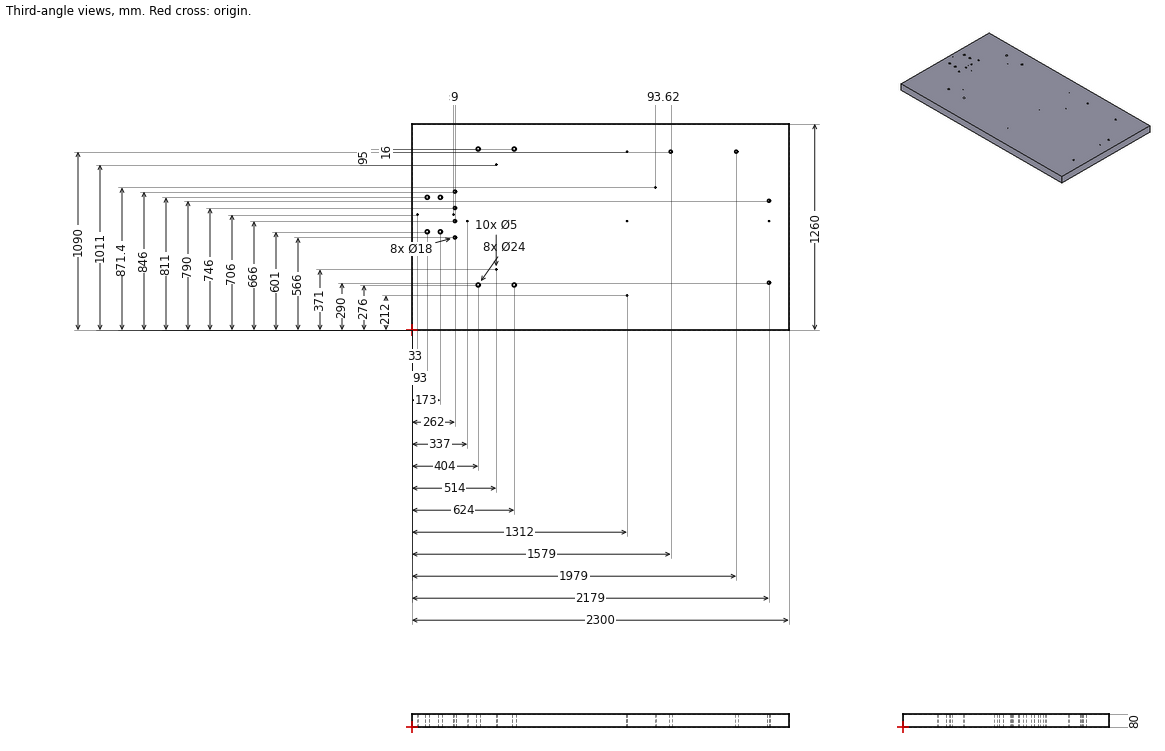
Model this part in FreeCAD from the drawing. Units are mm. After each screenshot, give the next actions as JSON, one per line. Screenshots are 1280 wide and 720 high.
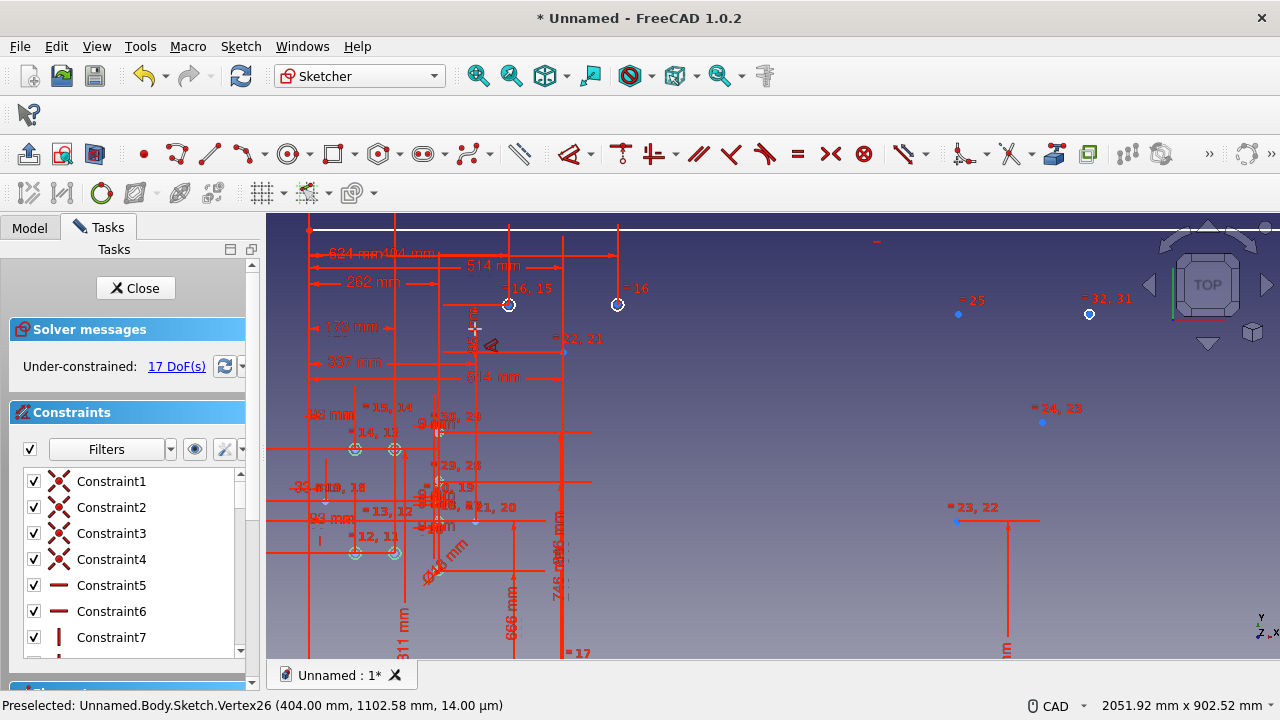
{"action": "left_click", "coordinate": [563, 352]}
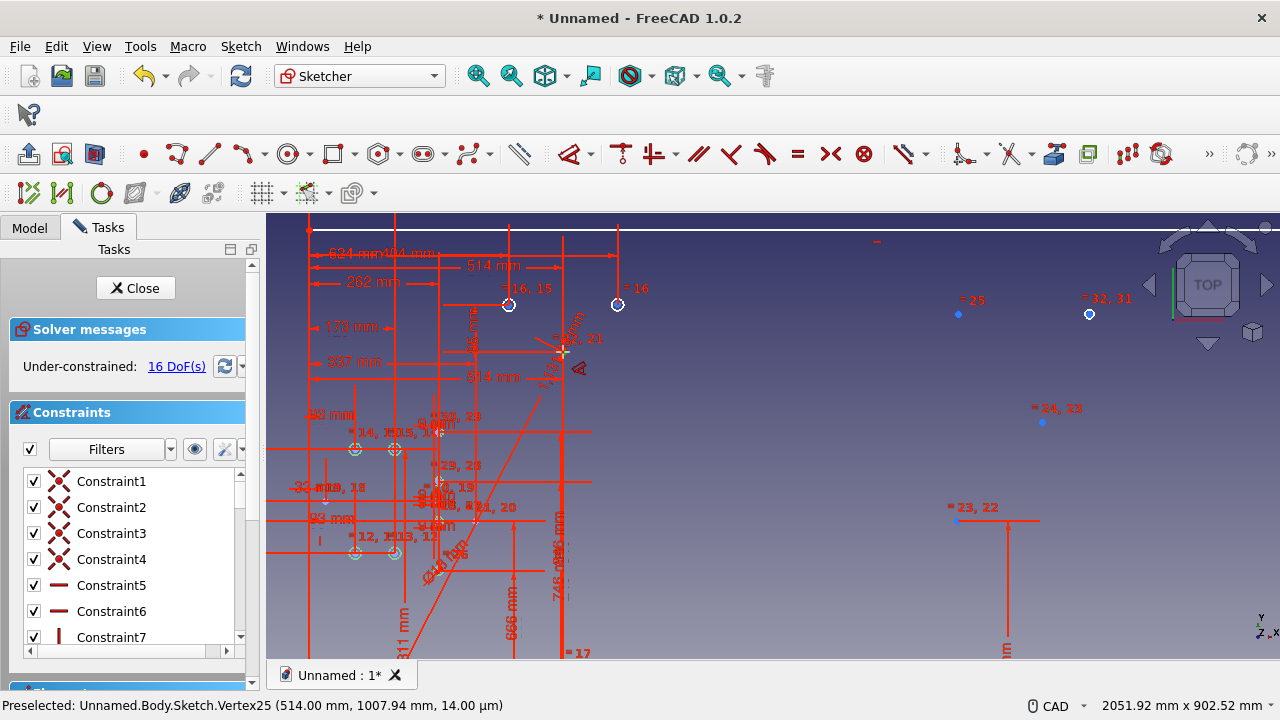
{"action": "left_click", "coordinate": [618, 305]}
{"action": "left_click", "coordinate": [652, 328]}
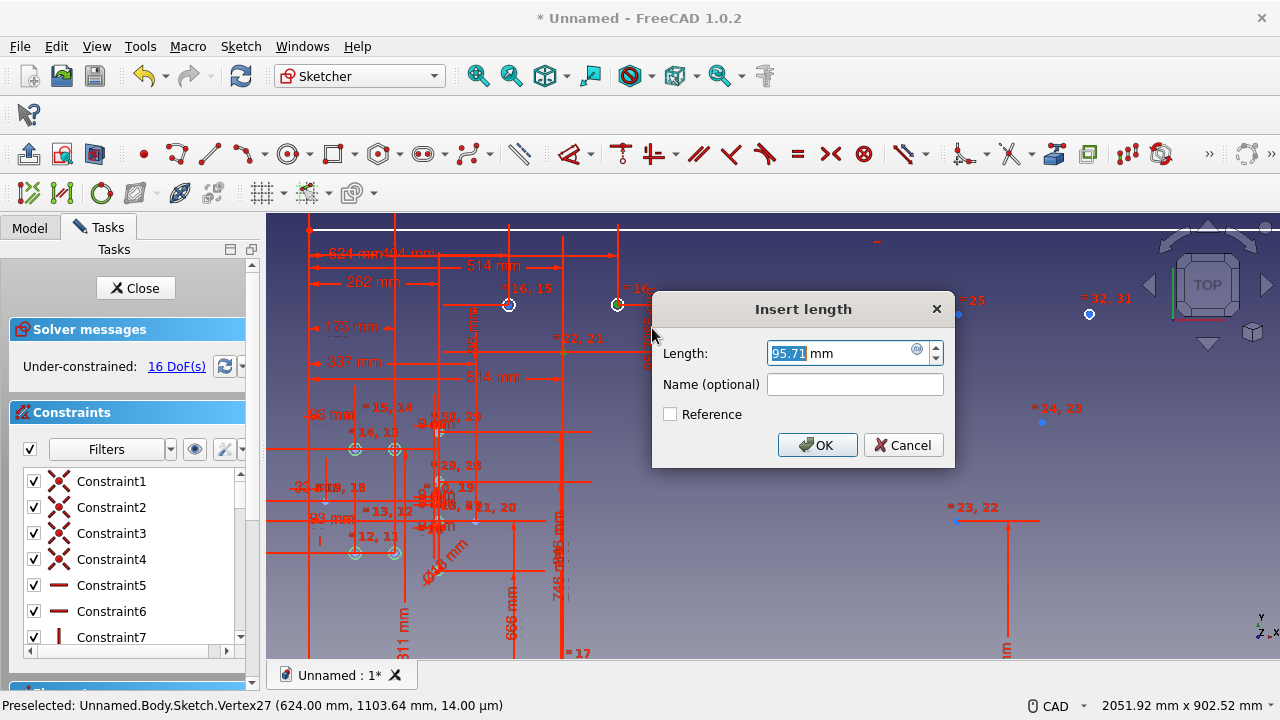
{"action": "type", "text": "95"}
{"action": "key", "text": "Return"}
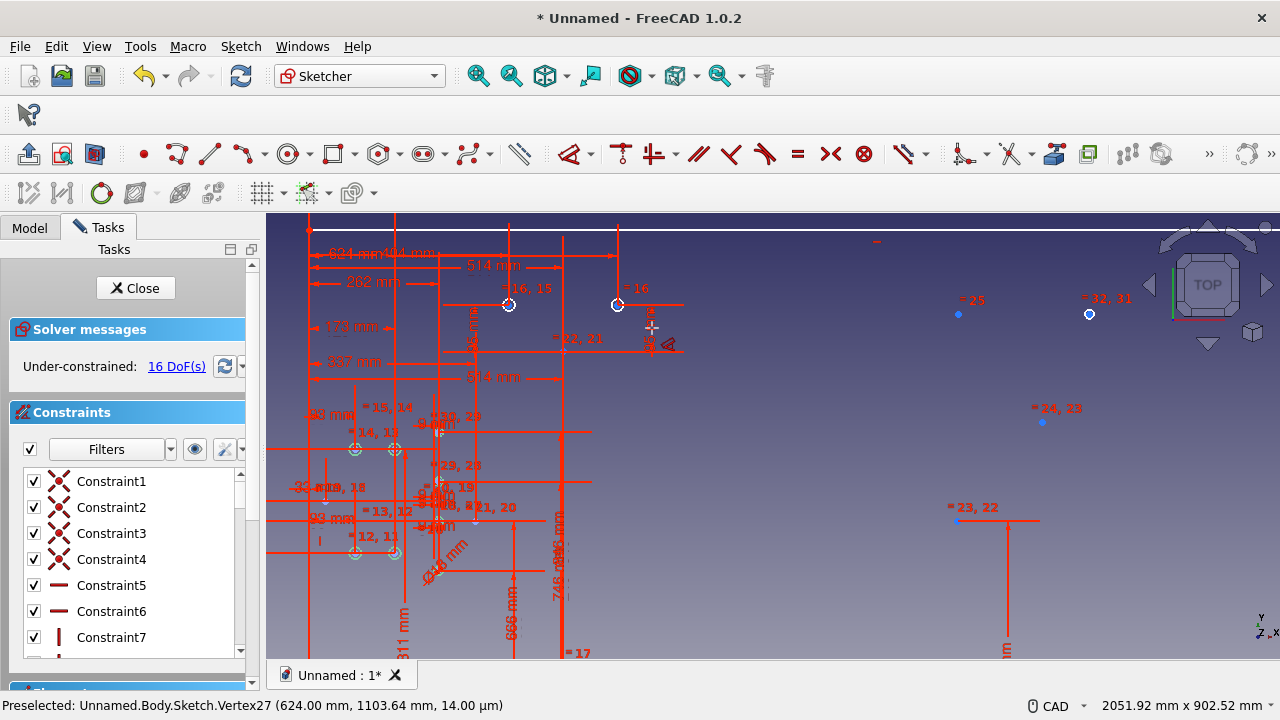
{"action": "scroll", "coordinate": [618, 305], "scroll_direction": "up", "scroll_amount": 9}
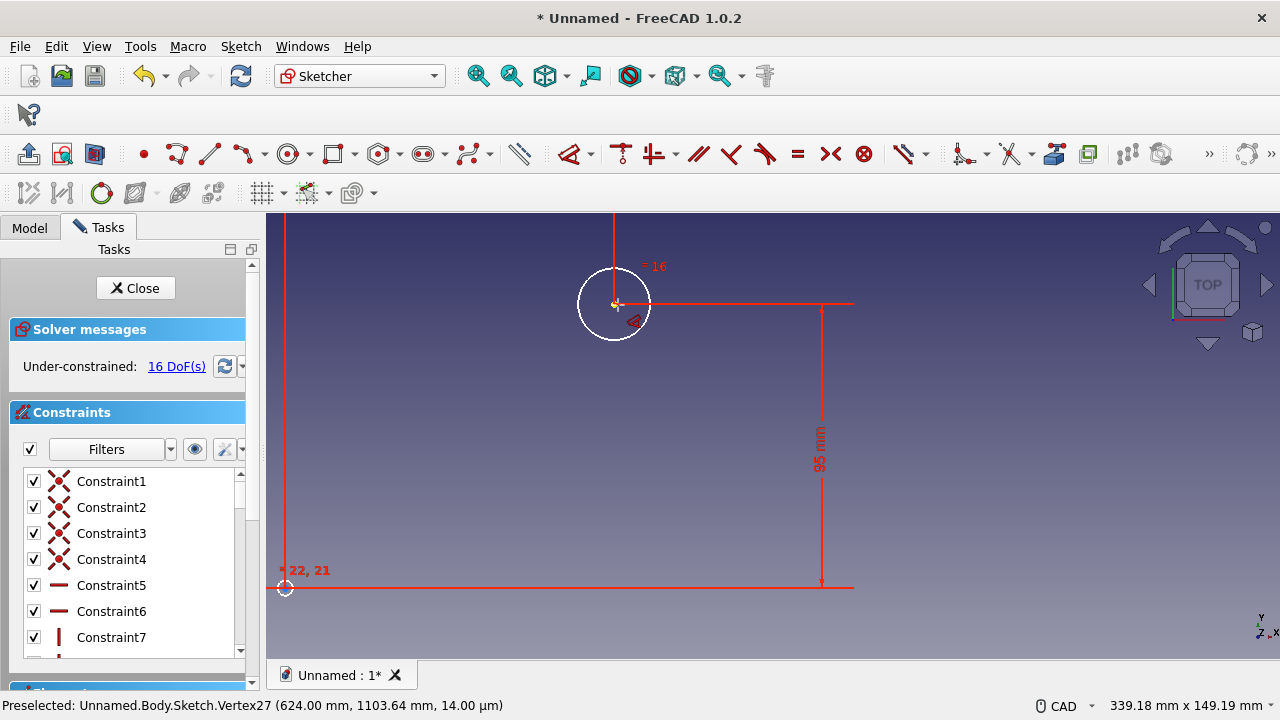
{"action": "left_click", "coordinate": [614, 304]}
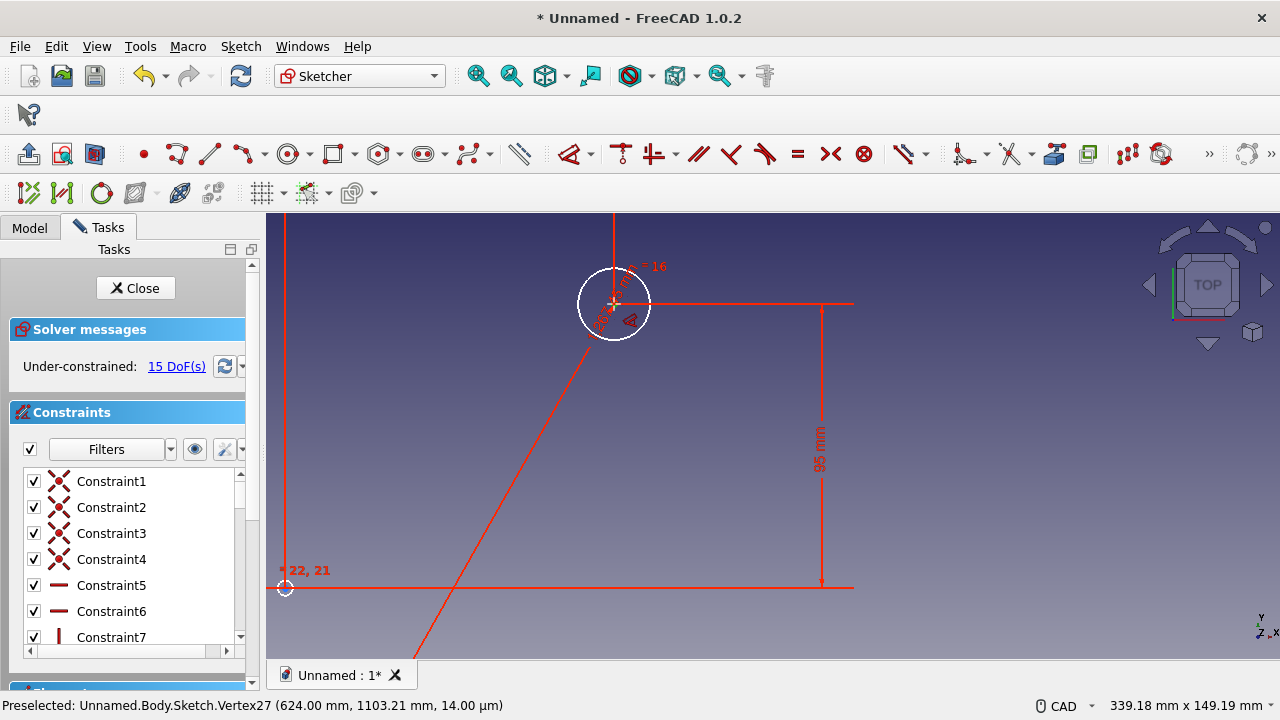
{"action": "scroll", "coordinate": [586, 333], "scroll_direction": "down", "scroll_amount": 13}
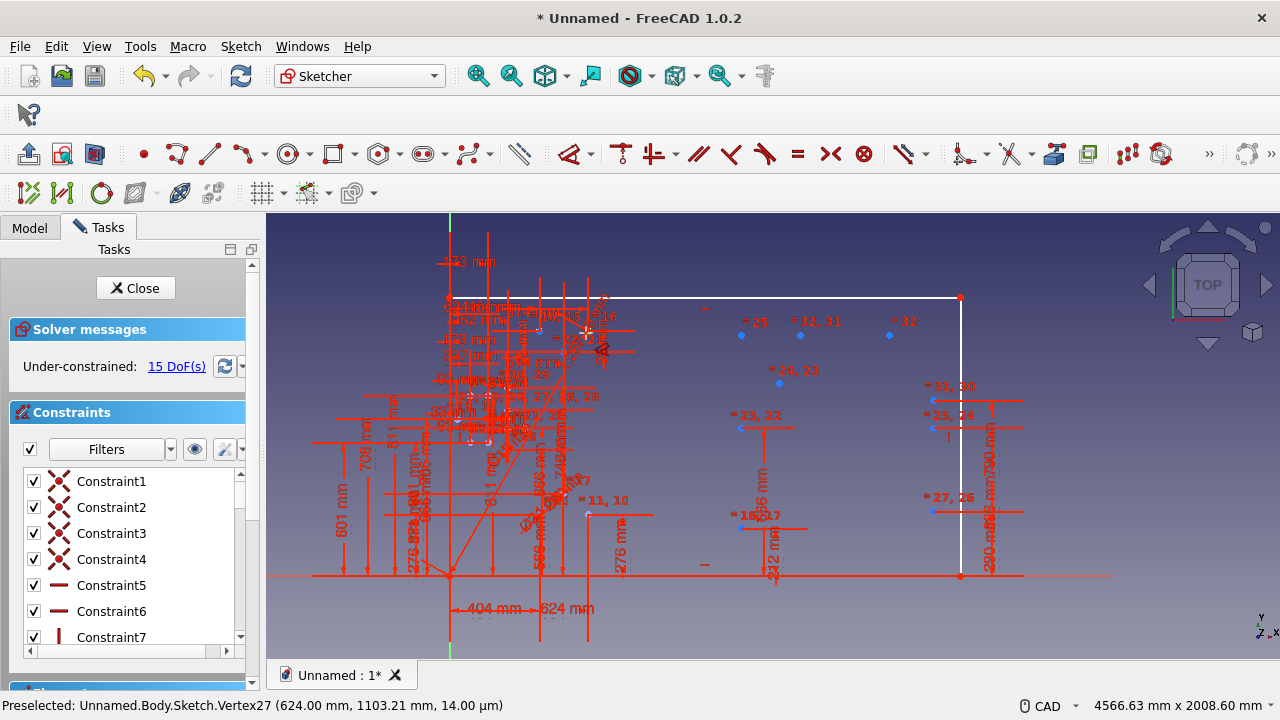
{"action": "scroll", "coordinate": [741, 335], "scroll_direction": "up", "scroll_amount": 13}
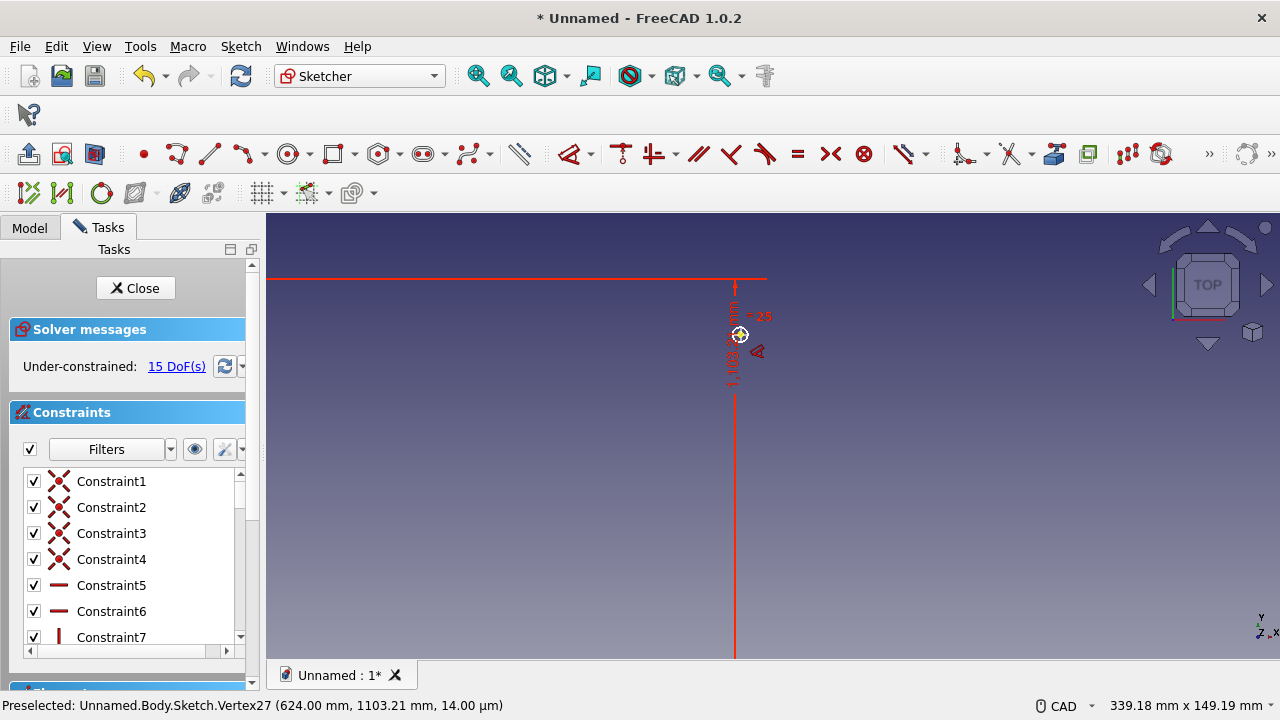
{"action": "left_click", "coordinate": [740, 335]}
{"action": "left_click", "coordinate": [774, 307]}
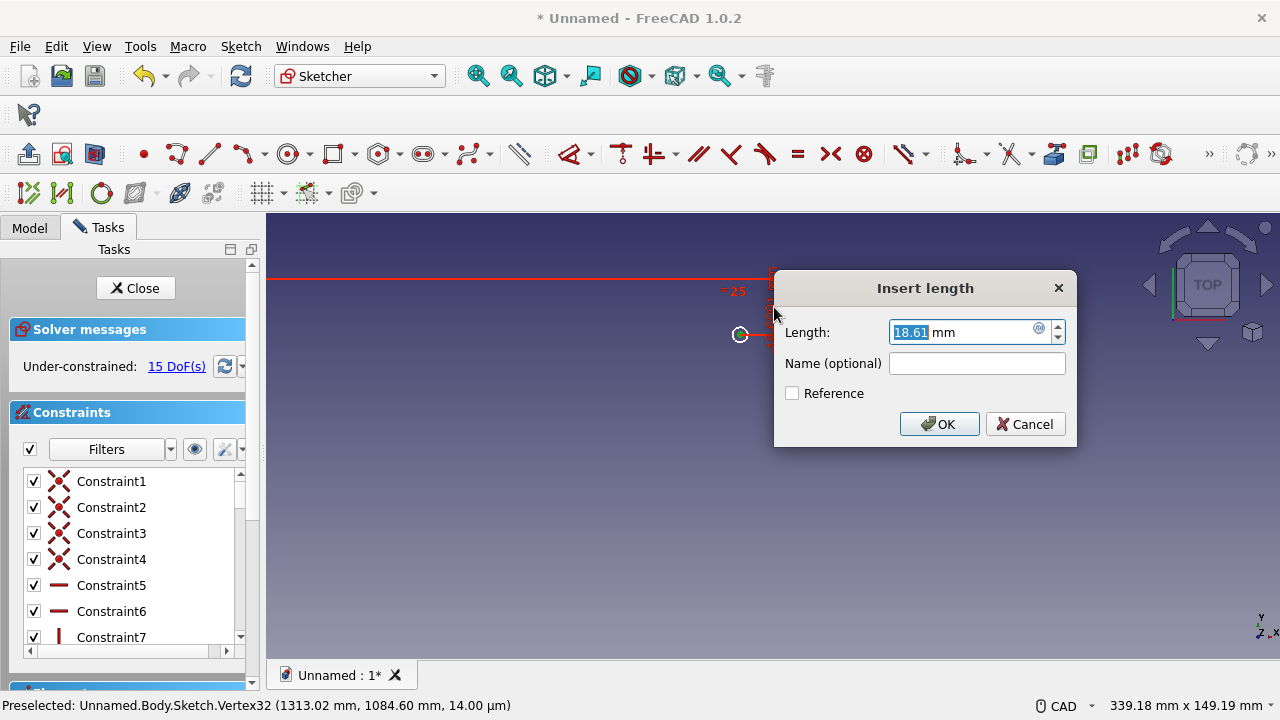
{"action": "type", "text": "16"}
{"action": "key", "text": "Return"}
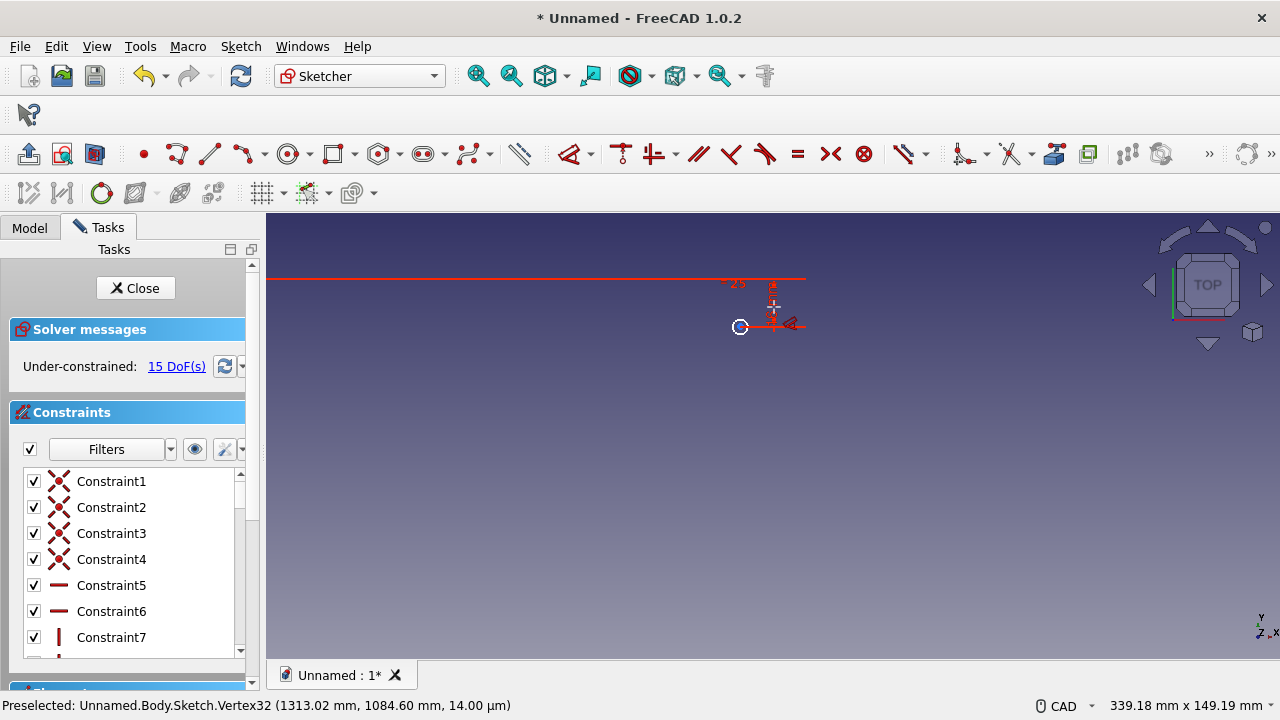
{"action": "scroll", "coordinate": [741, 335], "scroll_direction": "down", "scroll_amount": 13}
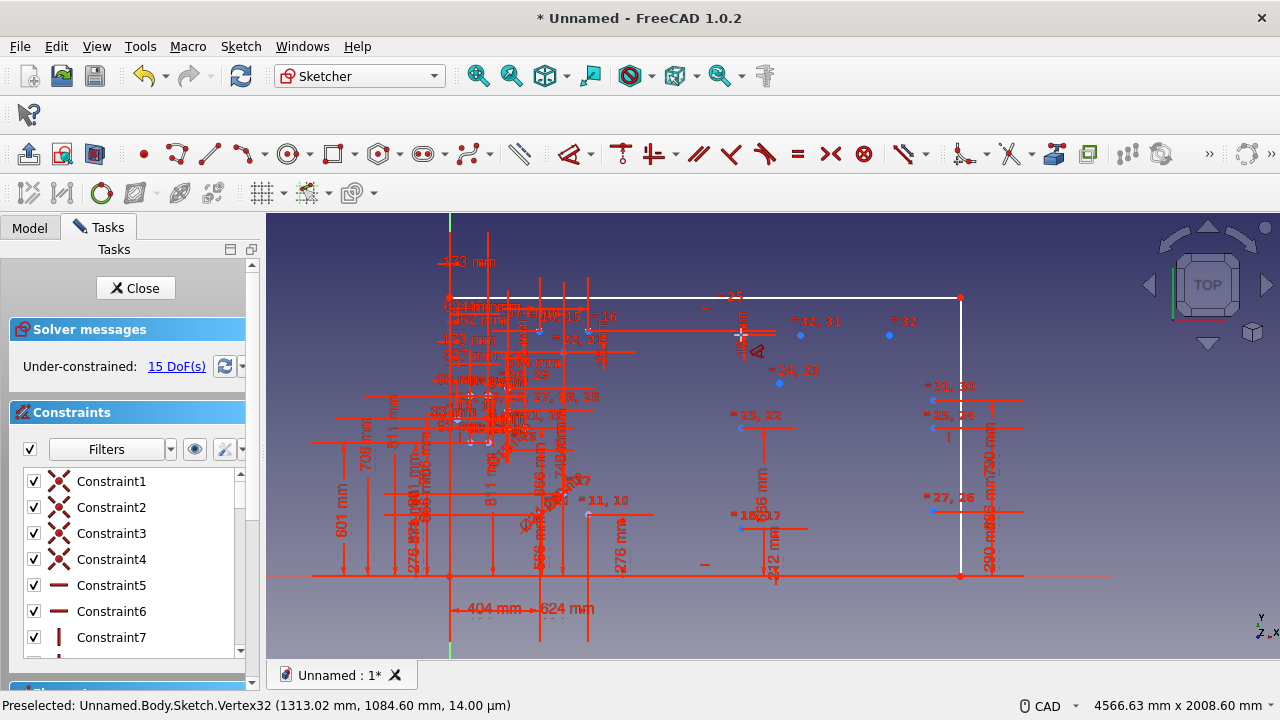
{"action": "left_click", "coordinate": [603, 576]}
{"action": "left_click", "coordinate": [705, 610]}